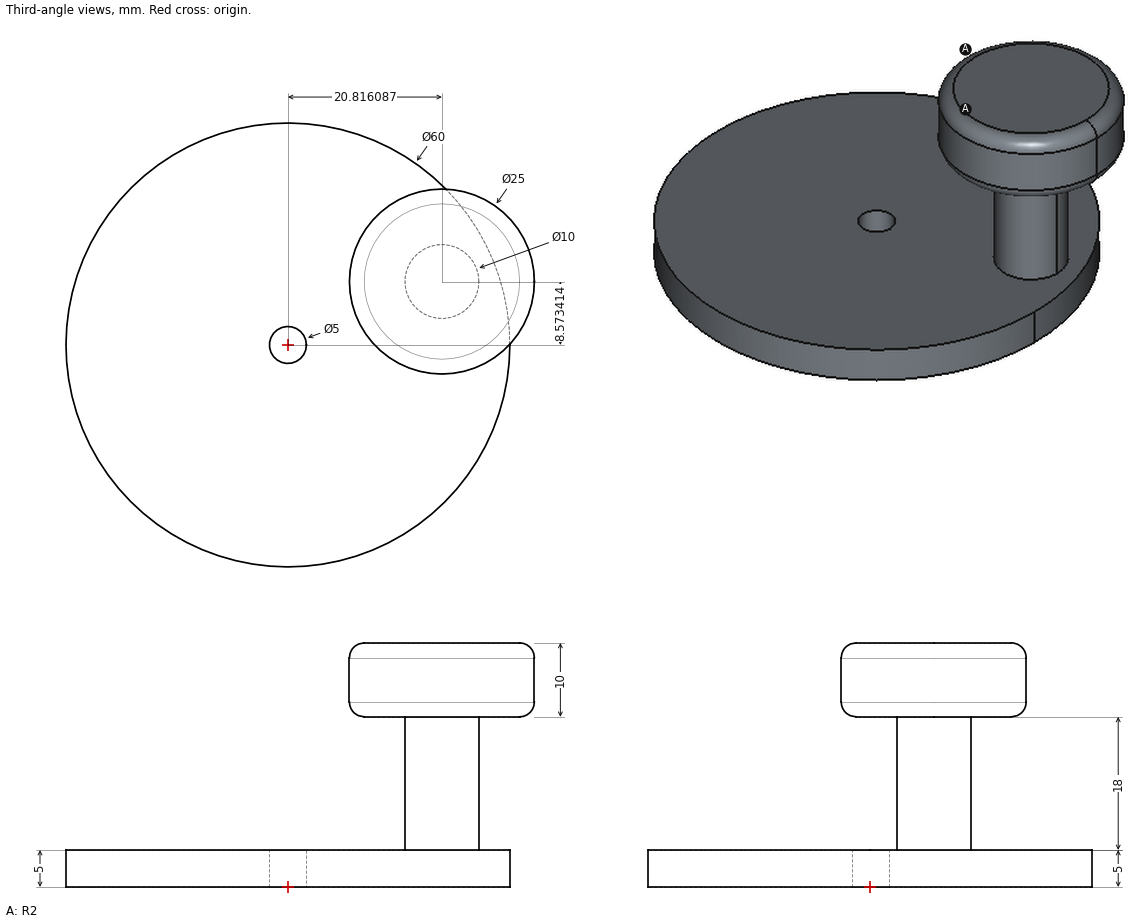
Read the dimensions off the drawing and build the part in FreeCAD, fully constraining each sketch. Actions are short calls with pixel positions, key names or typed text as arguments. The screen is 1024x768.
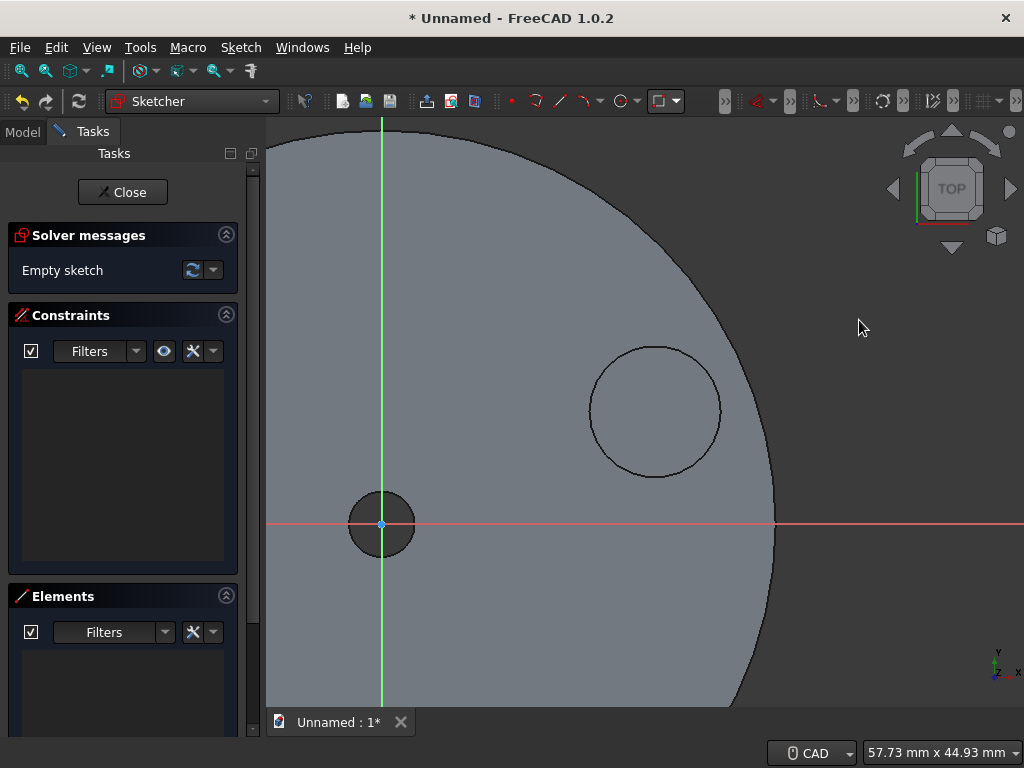
click(622, 102)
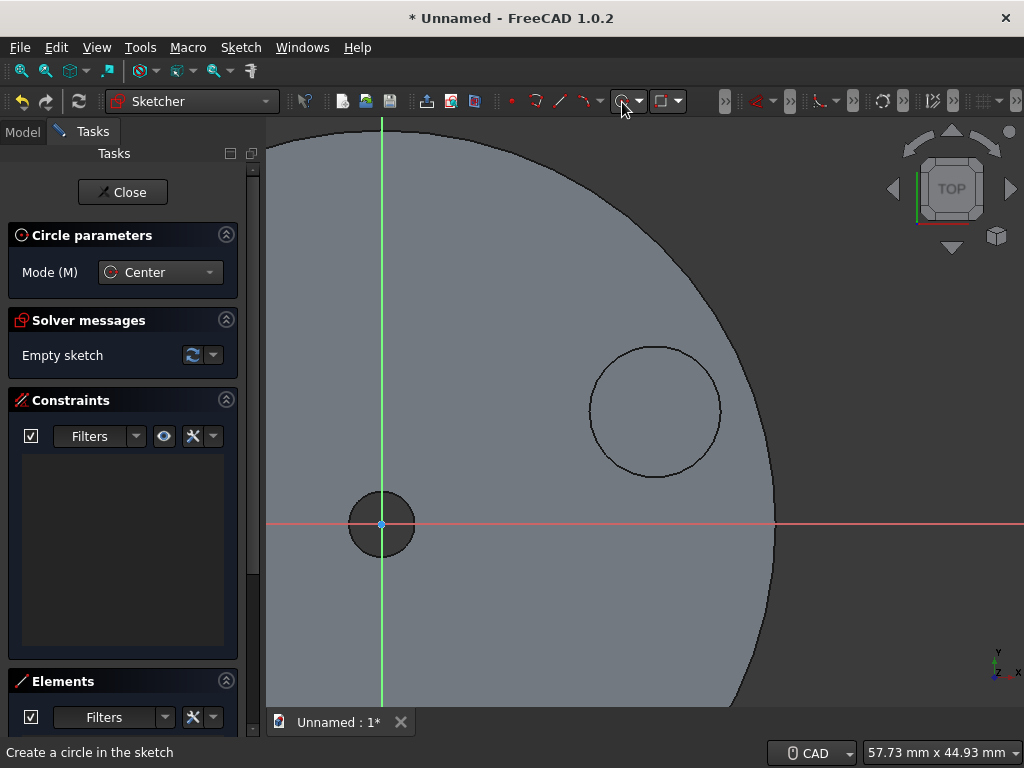
click(655, 412)
move(771, 296)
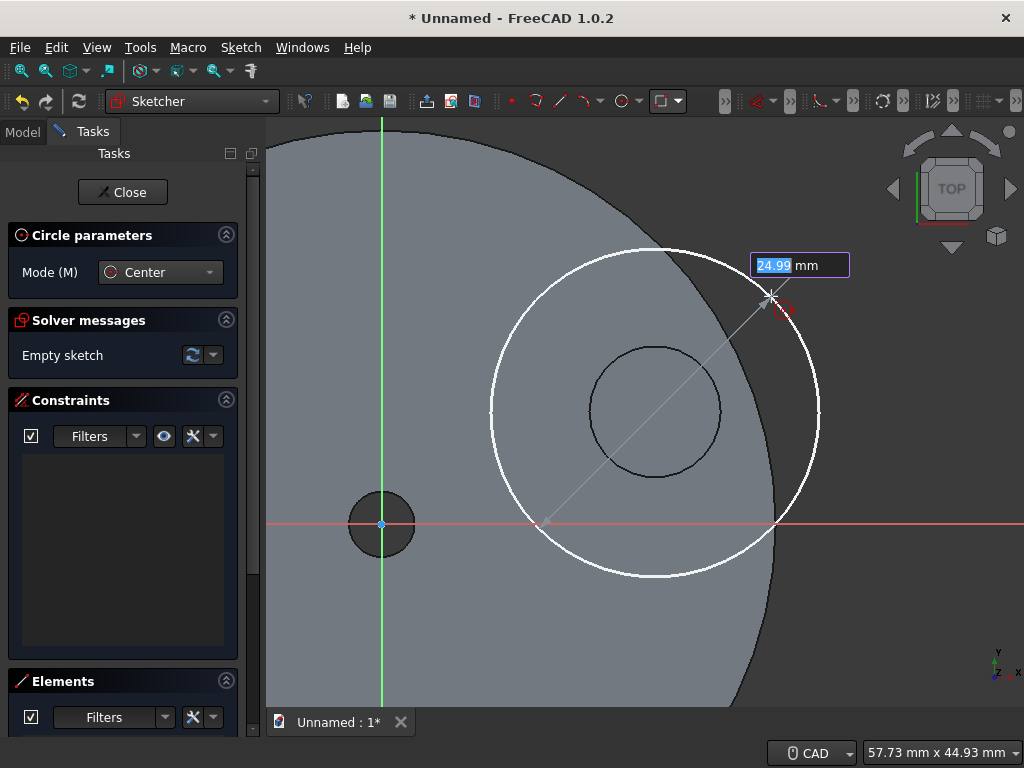
text(25)
key(Return)
key(Escape)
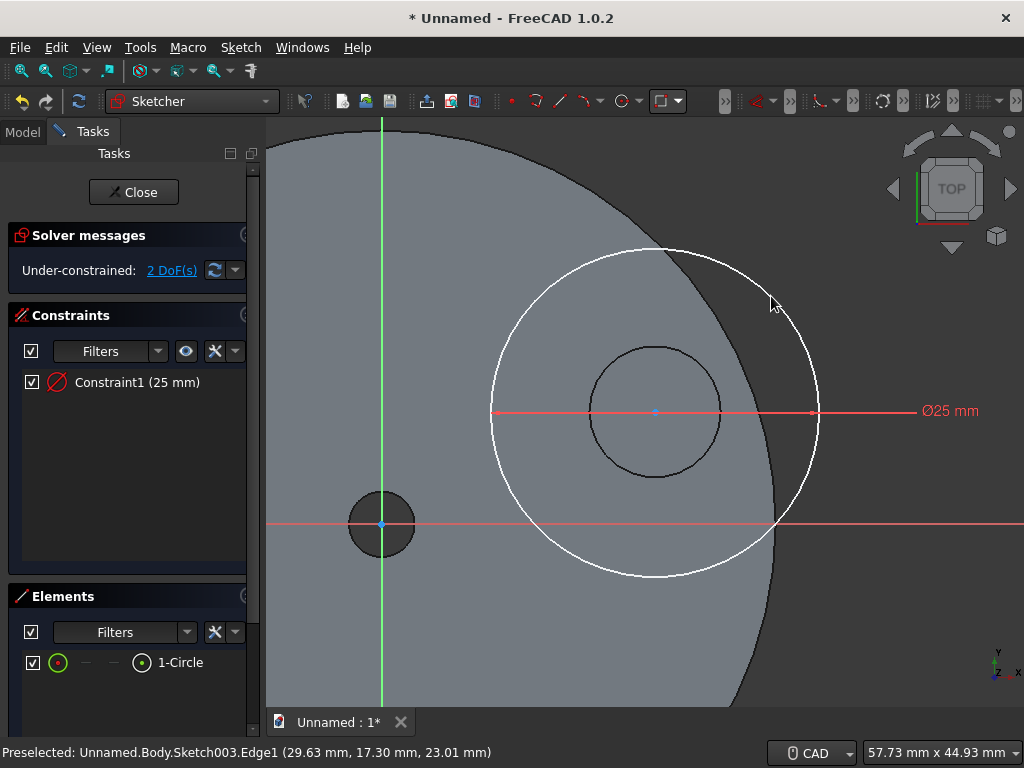
click(756, 102)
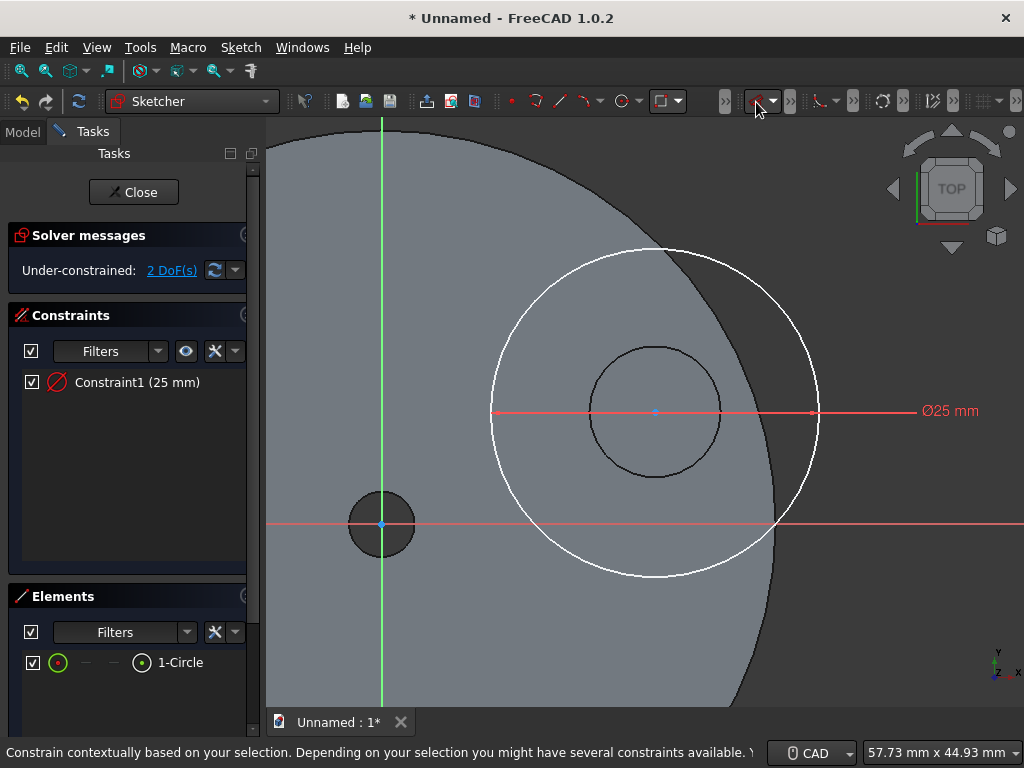
click(655, 413)
click(348, 469)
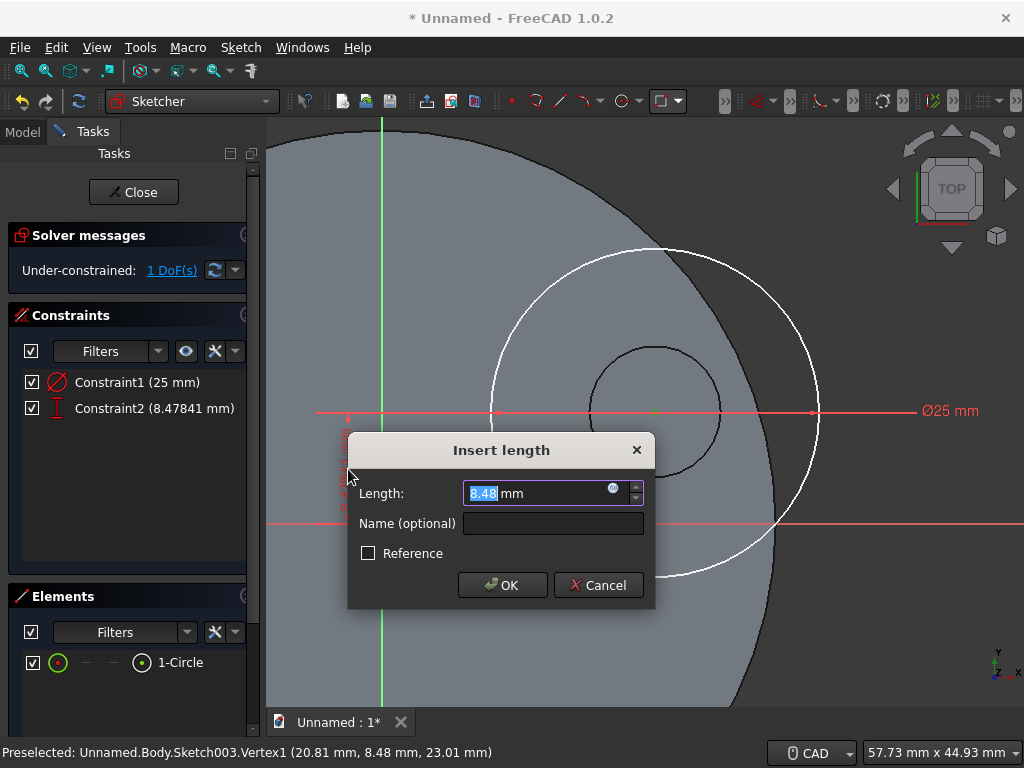
text(8.573414)
key(Return)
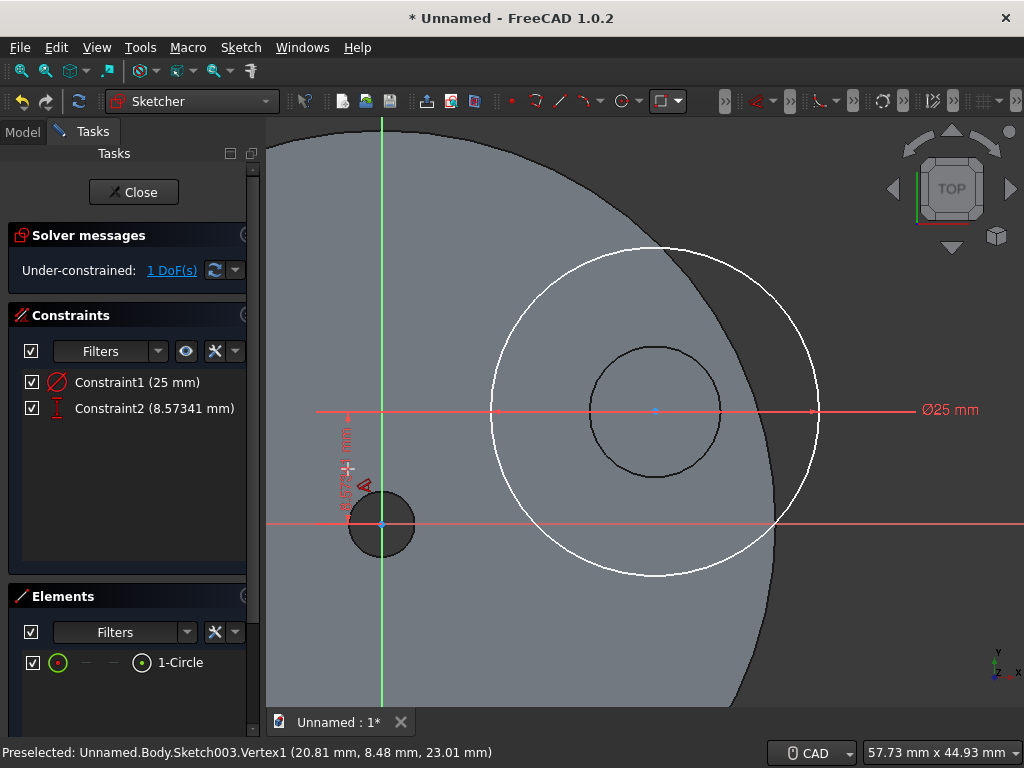
click(655, 412)
click(518, 558)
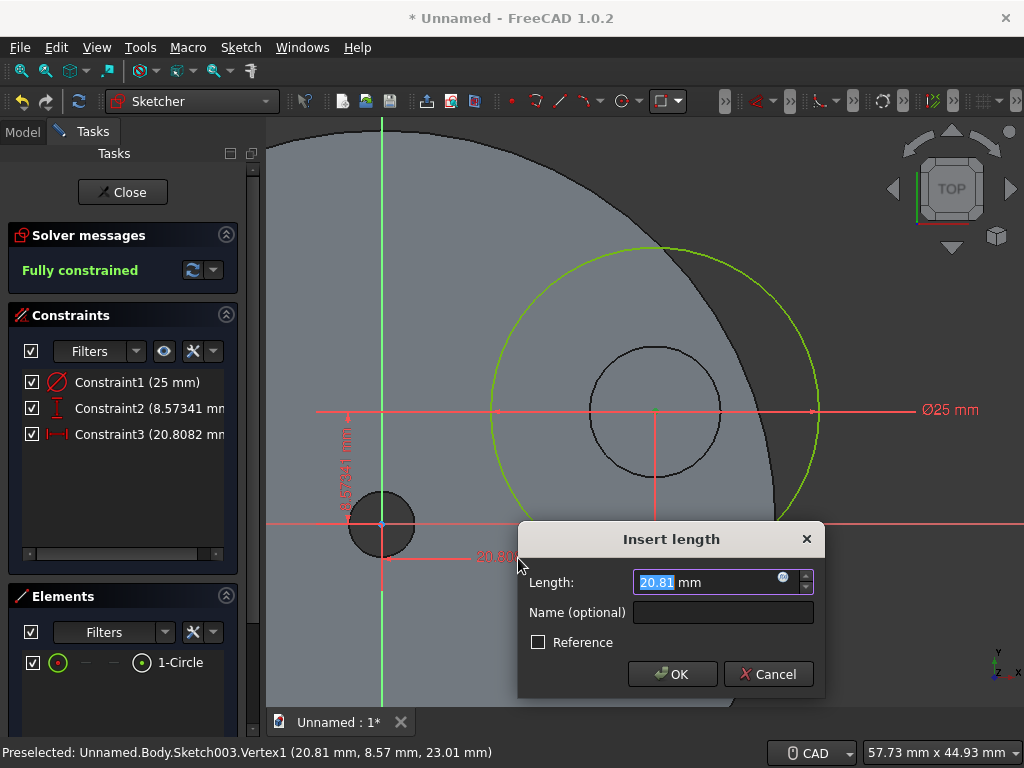
text(20.816087)
key(Return)
key(Escape)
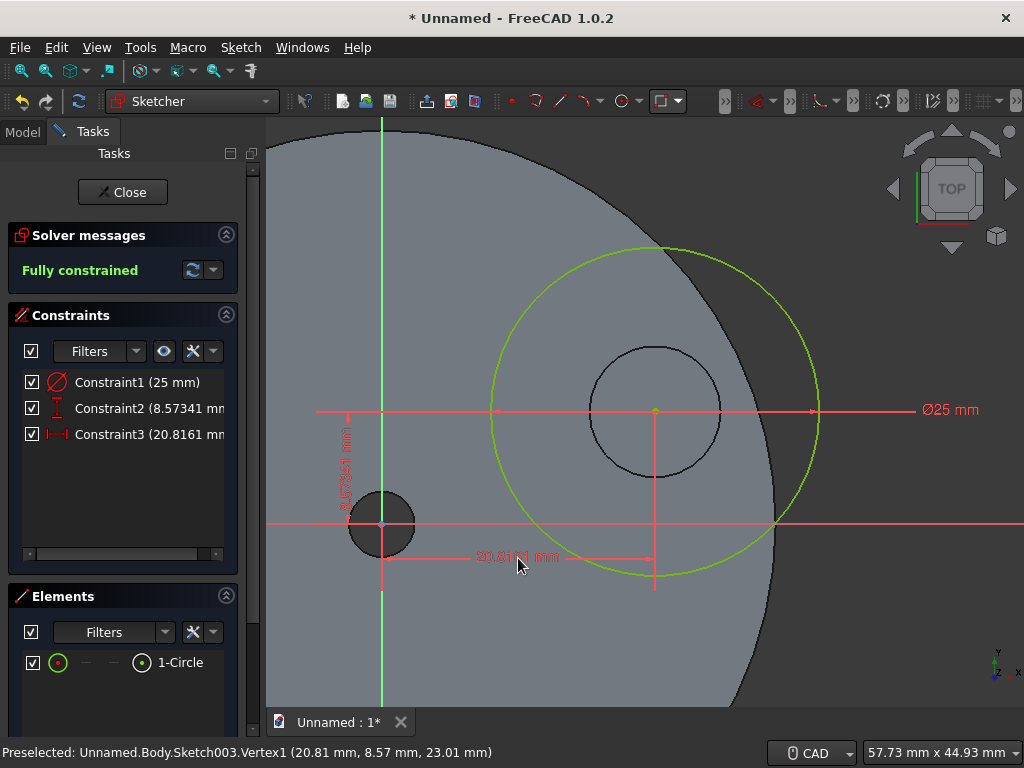
click(123, 192)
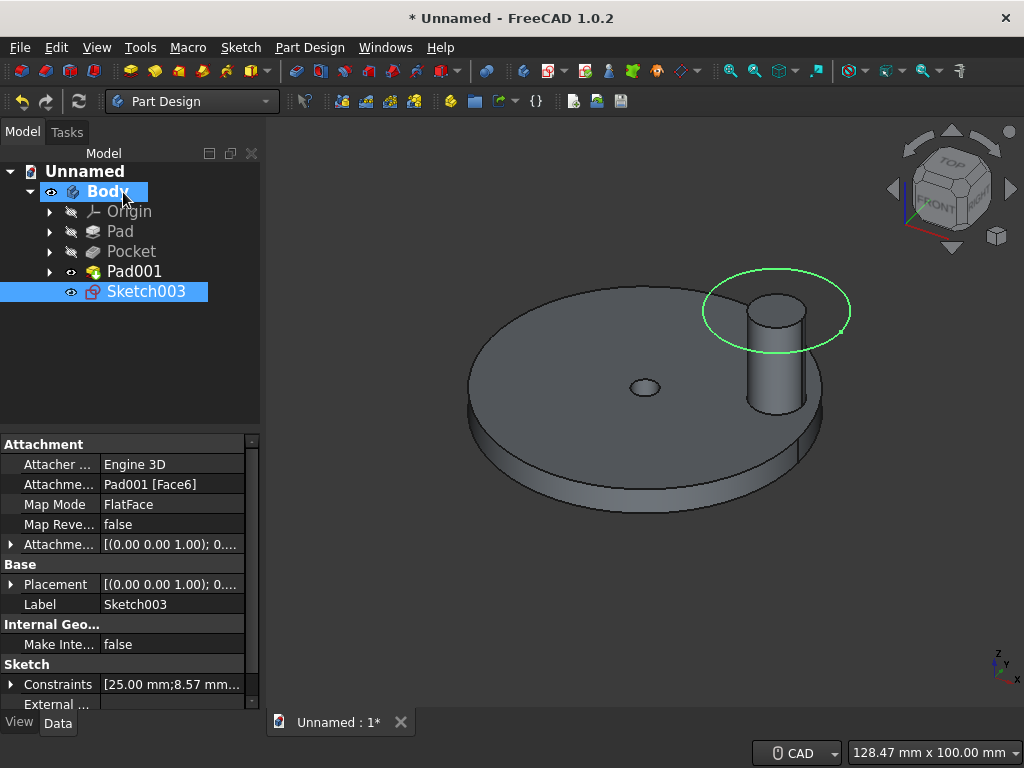
click(132, 72)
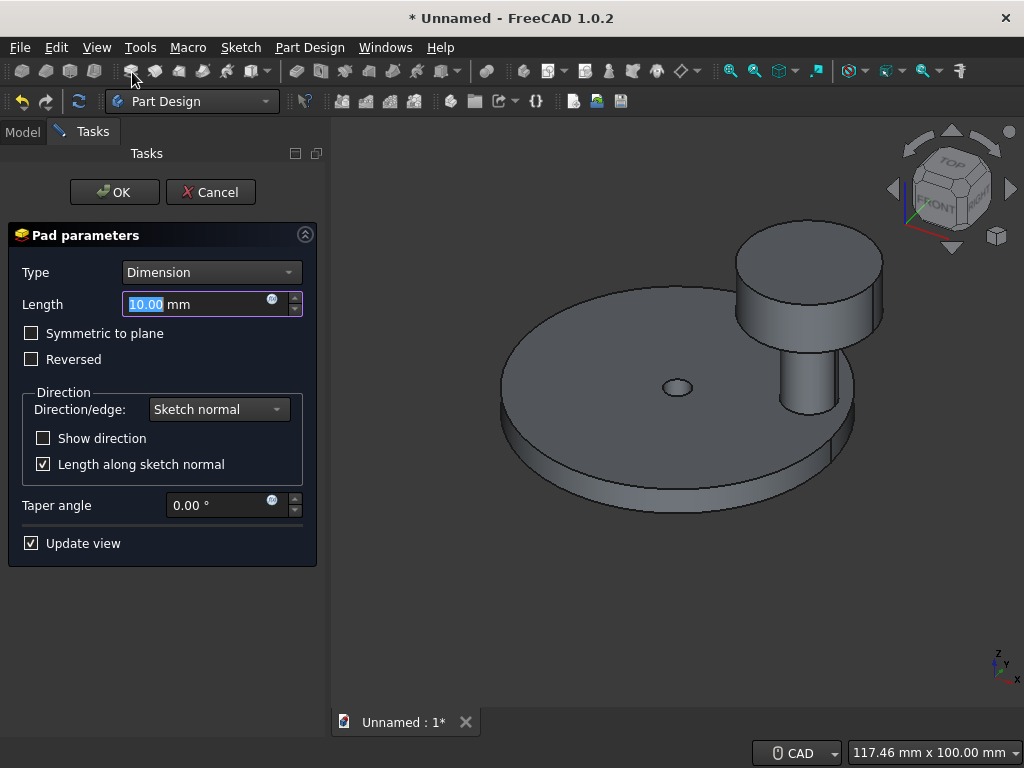
text(10)
key(Tab)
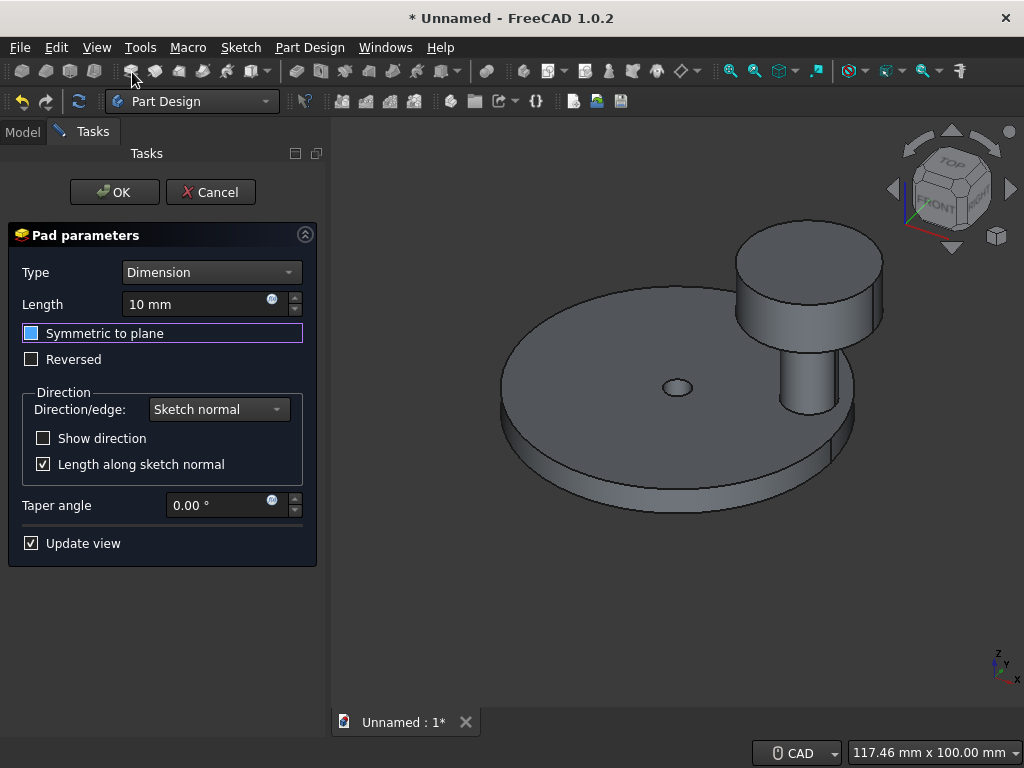
click(115, 192)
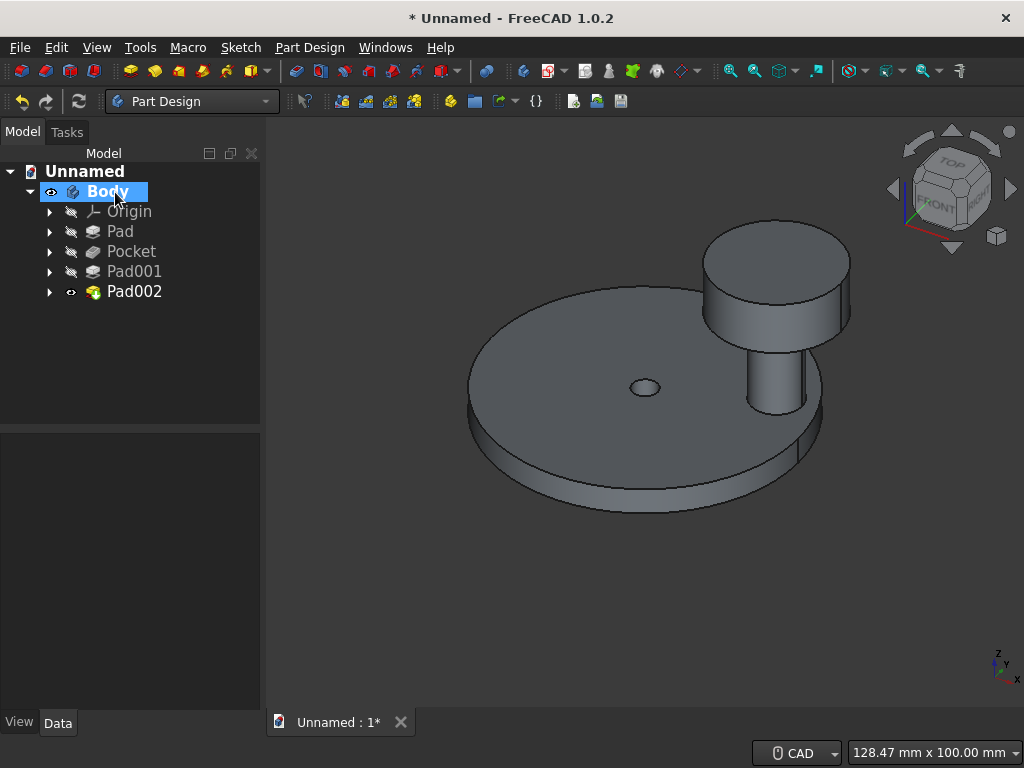
click(732, 72)